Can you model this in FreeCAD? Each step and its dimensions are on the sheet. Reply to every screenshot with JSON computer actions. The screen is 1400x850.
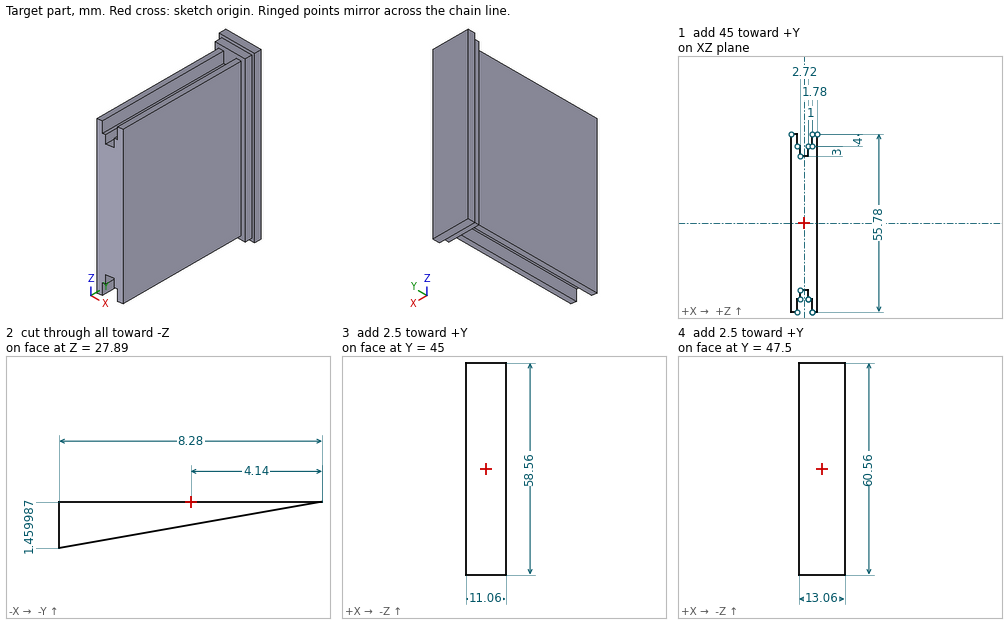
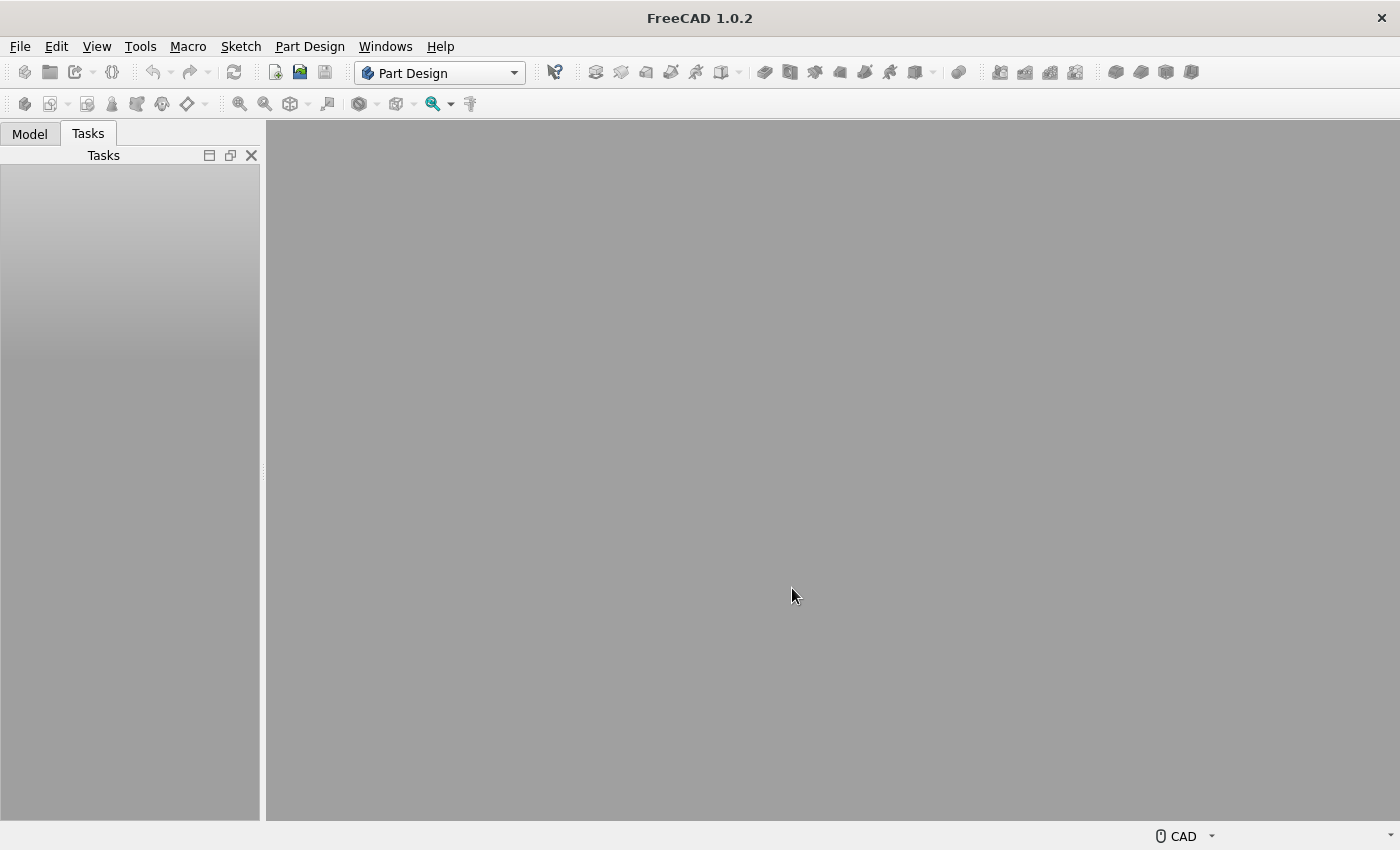
{"action": "left_click", "coordinate": [275, 72]}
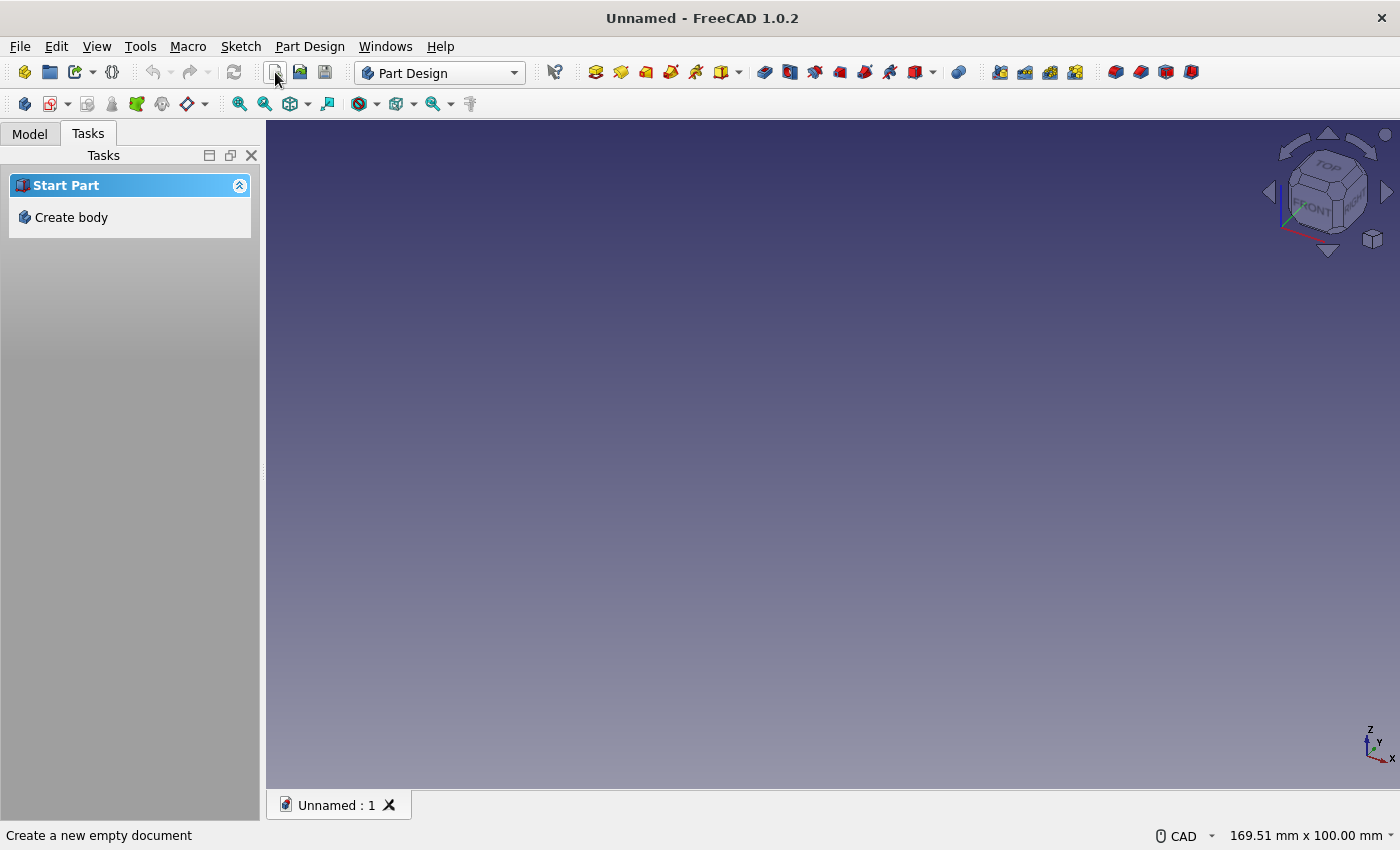
{"action": "left_click", "coordinate": [50, 104]}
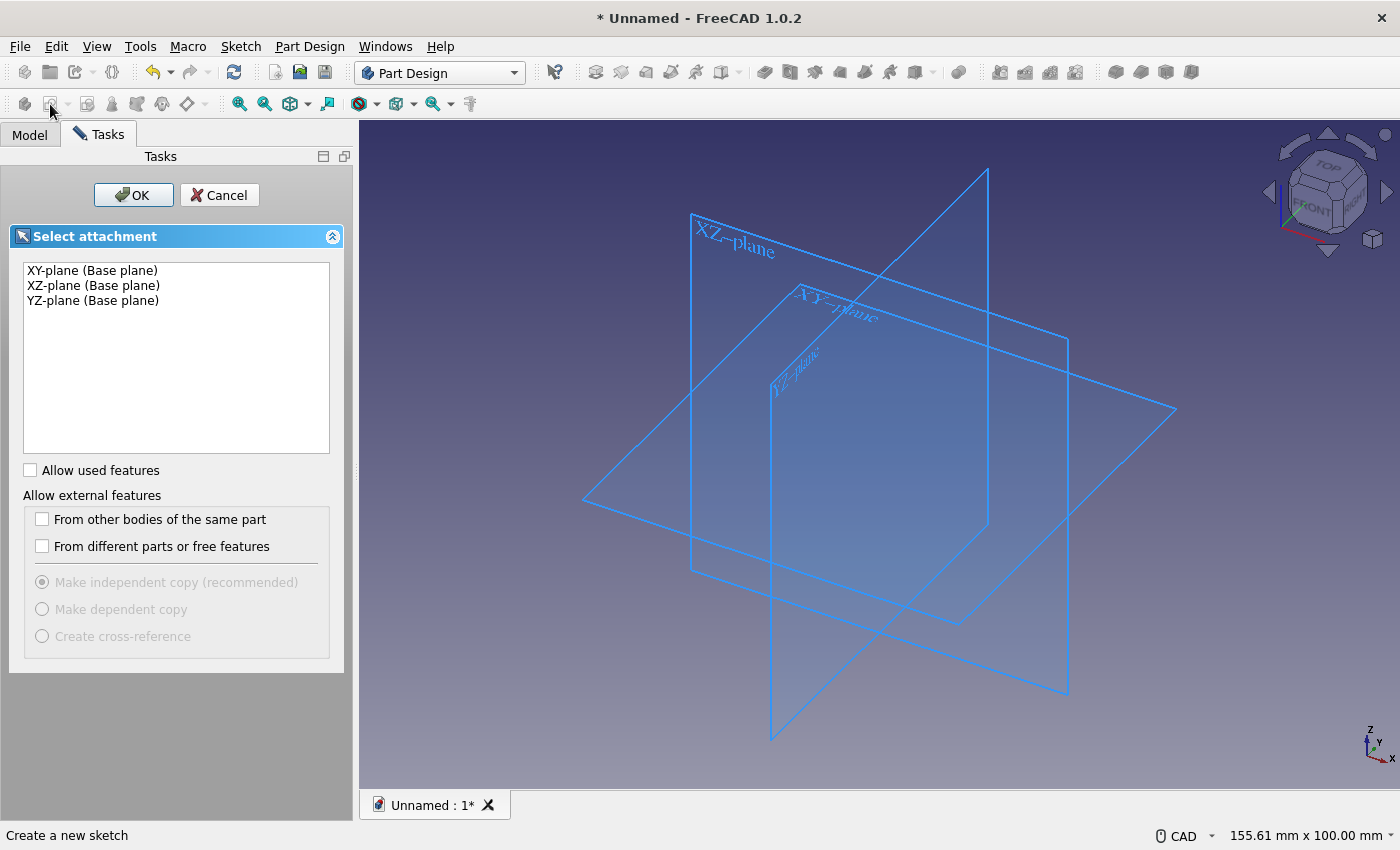
{"action": "left_click", "coordinate": [84, 286]}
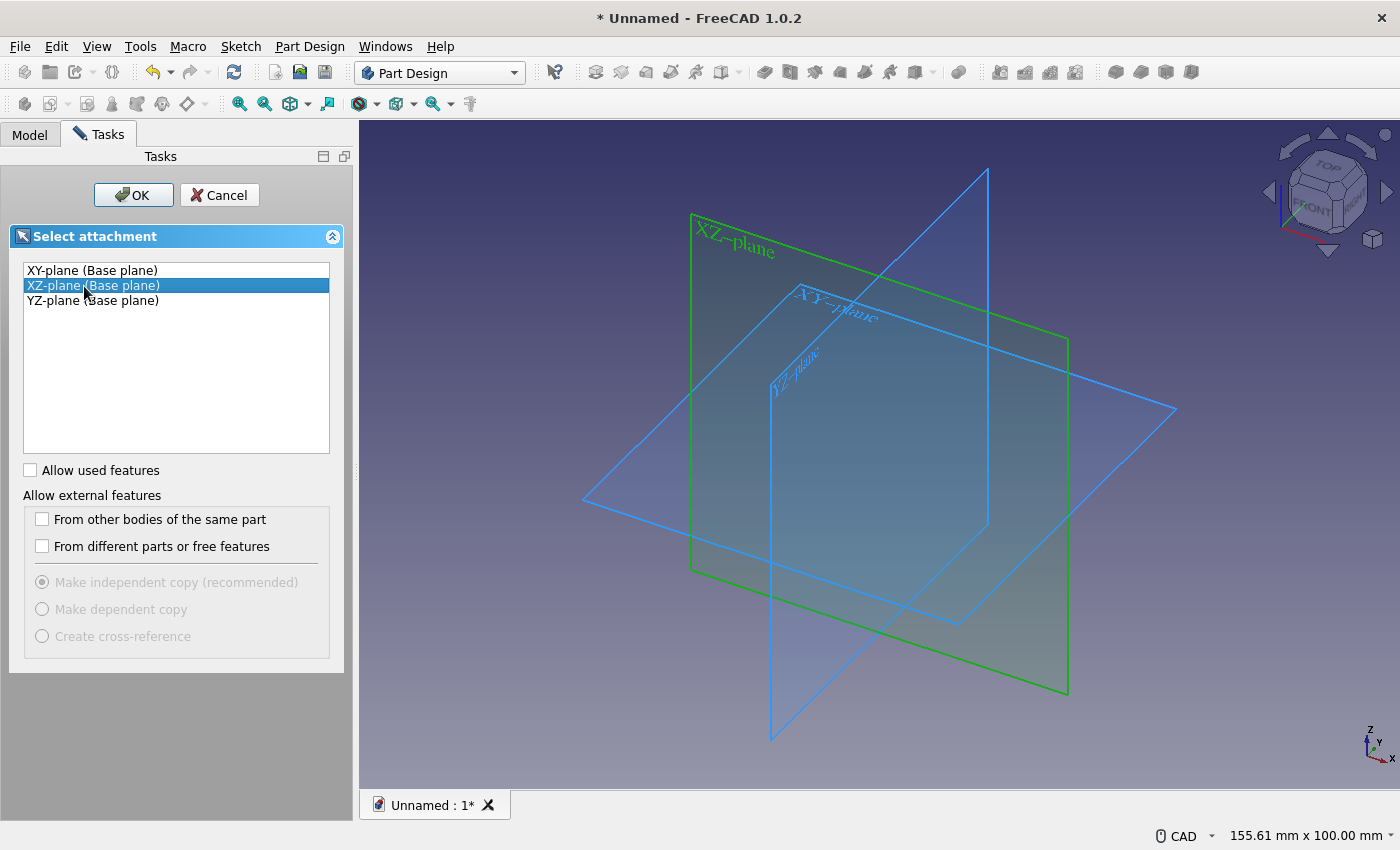
{"action": "left_click", "coordinate": [134, 195]}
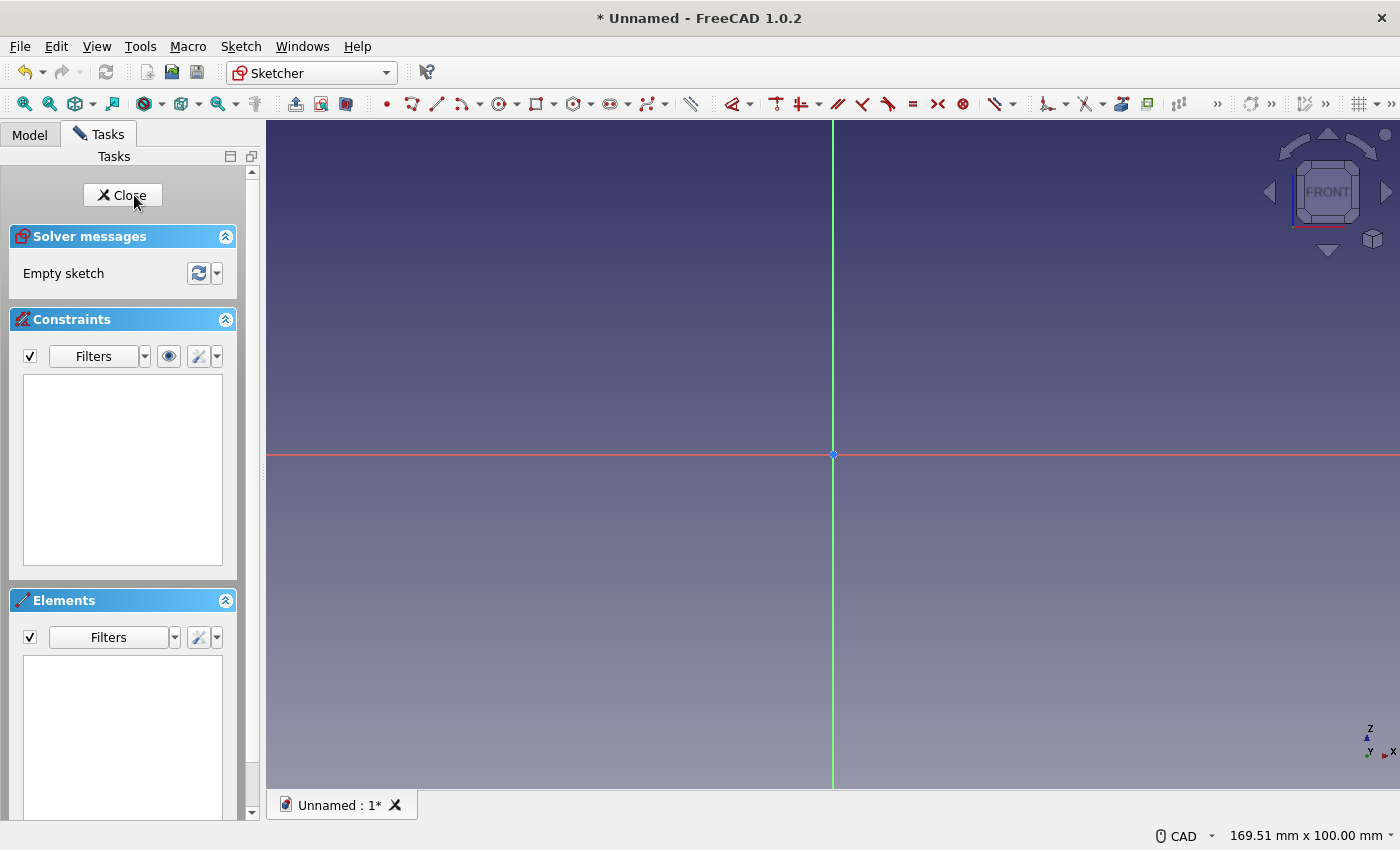
{"action": "left_click", "coordinate": [412, 104]}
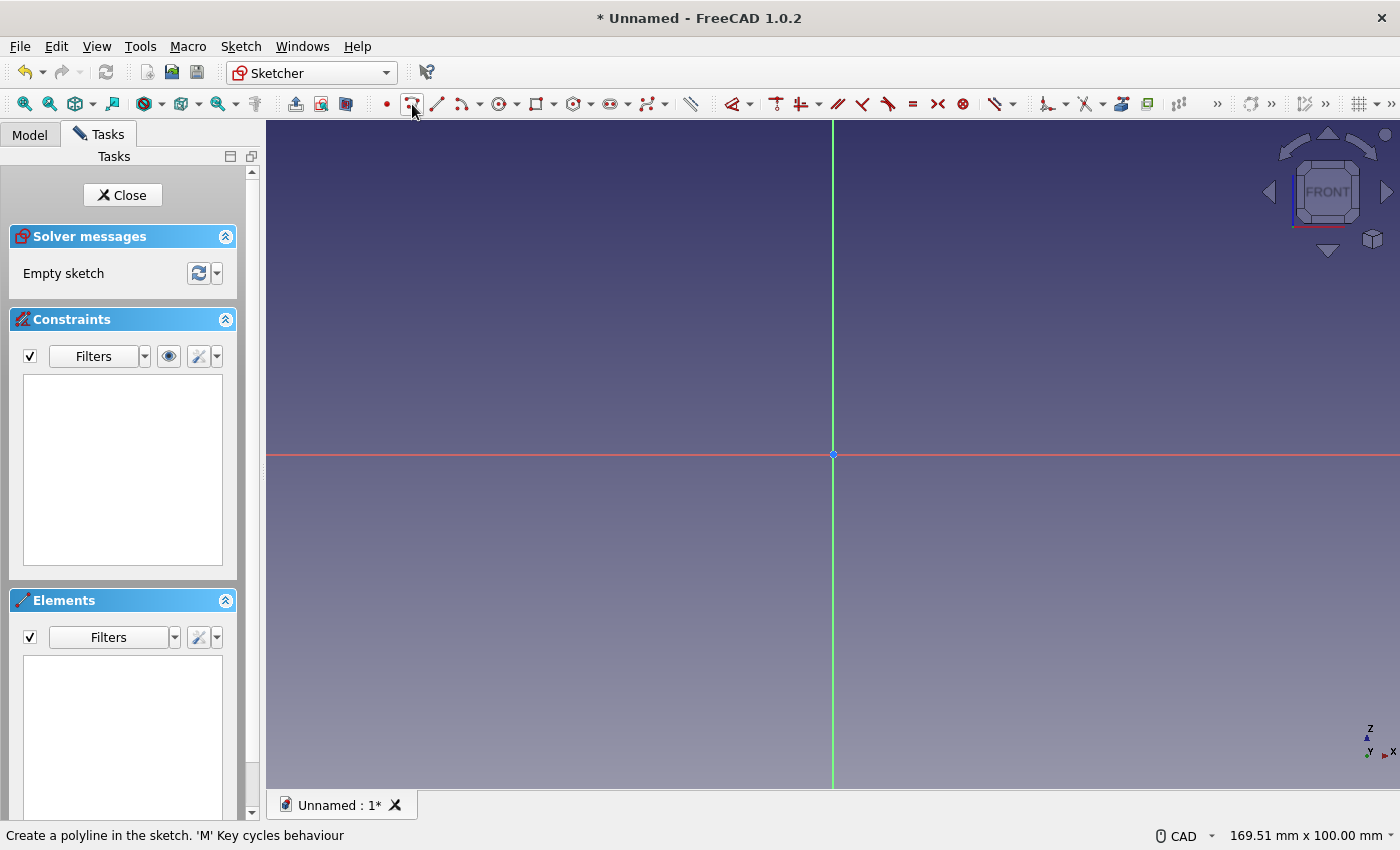
{"action": "scroll", "coordinate": [824, 315], "scroll_direction": "up", "scroll_amount": 3}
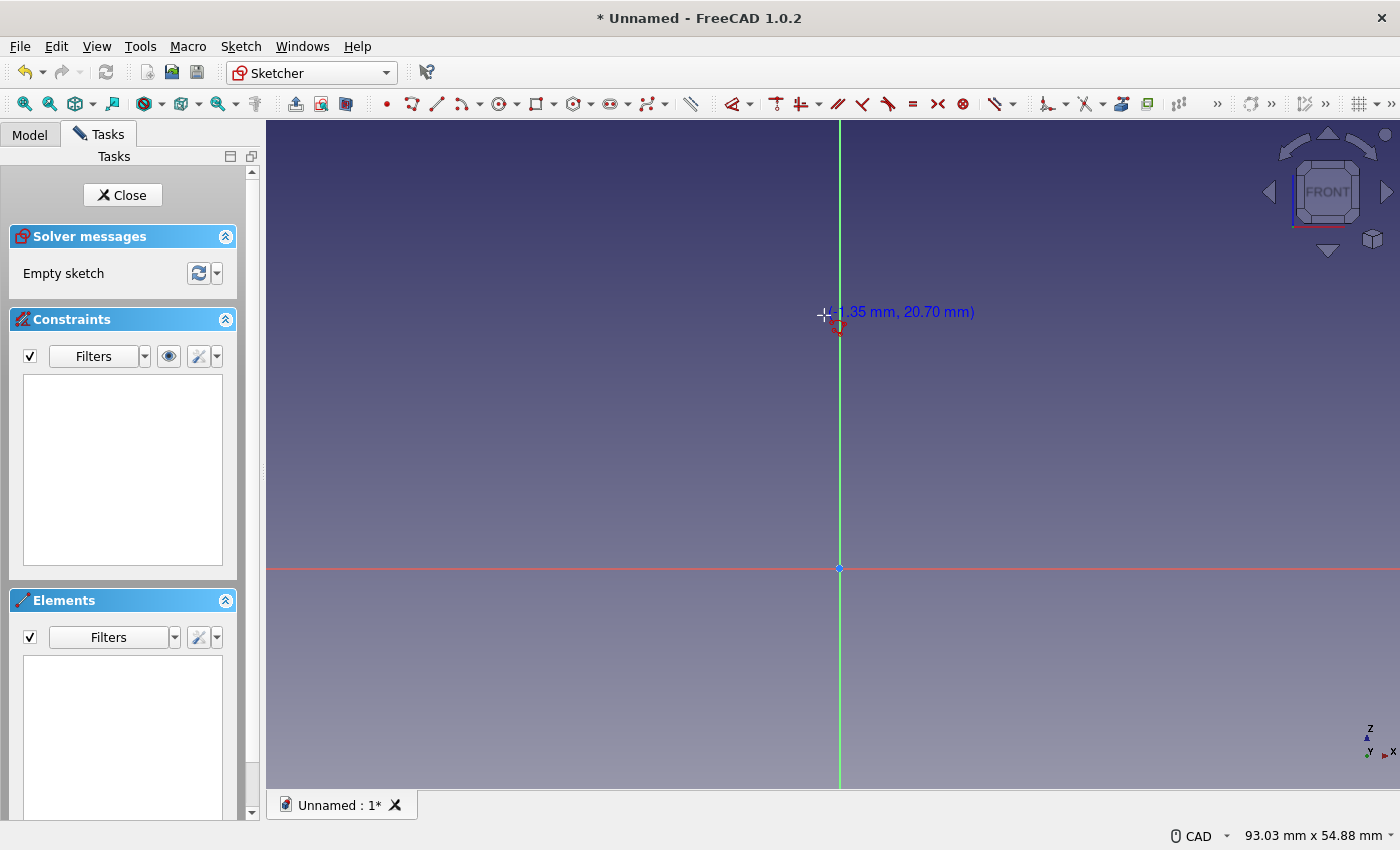
{"action": "left_click", "coordinate": [823, 314]}
{"action": "left_click", "coordinate": [857, 314]}
{"action": "left_click", "coordinate": [857, 278]}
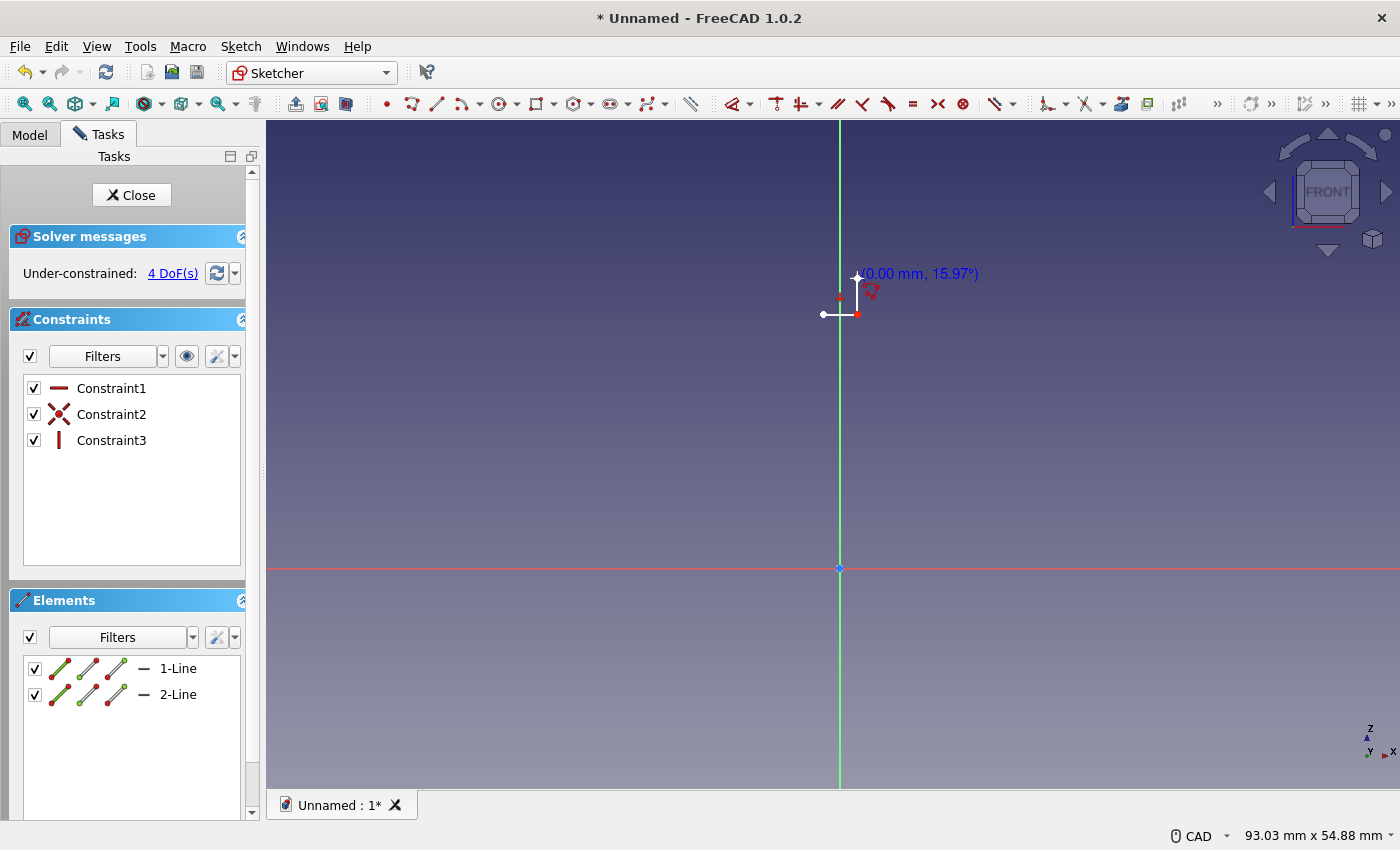
{"action": "scroll", "coordinate": [869, 278], "scroll_direction": "up", "scroll_amount": 2}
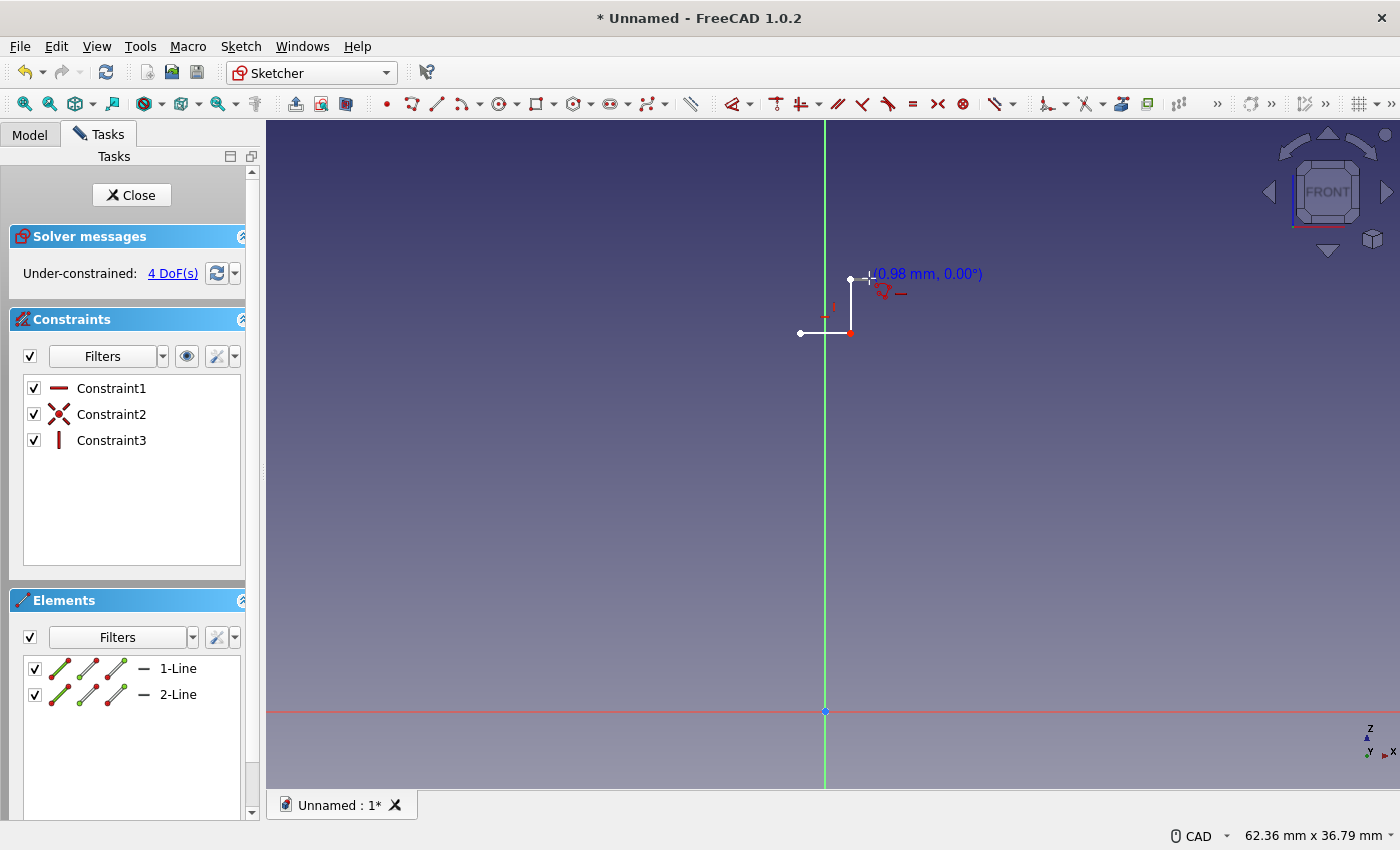
{"action": "left_click", "coordinate": [868, 278]}
{"action": "left_click", "coordinate": [868, 205]}
{"action": "left_click", "coordinate": [901, 205]}